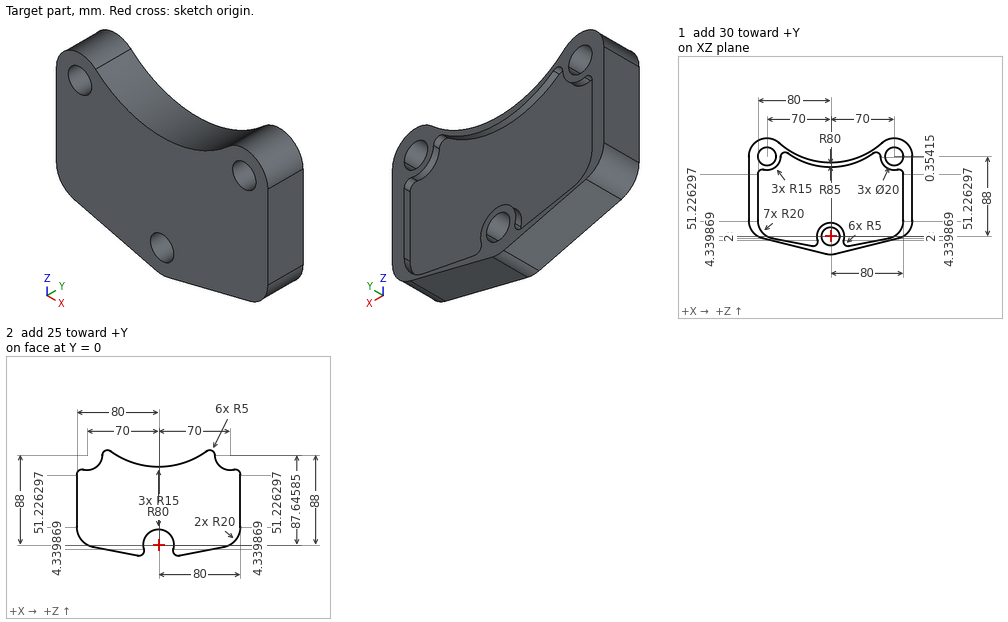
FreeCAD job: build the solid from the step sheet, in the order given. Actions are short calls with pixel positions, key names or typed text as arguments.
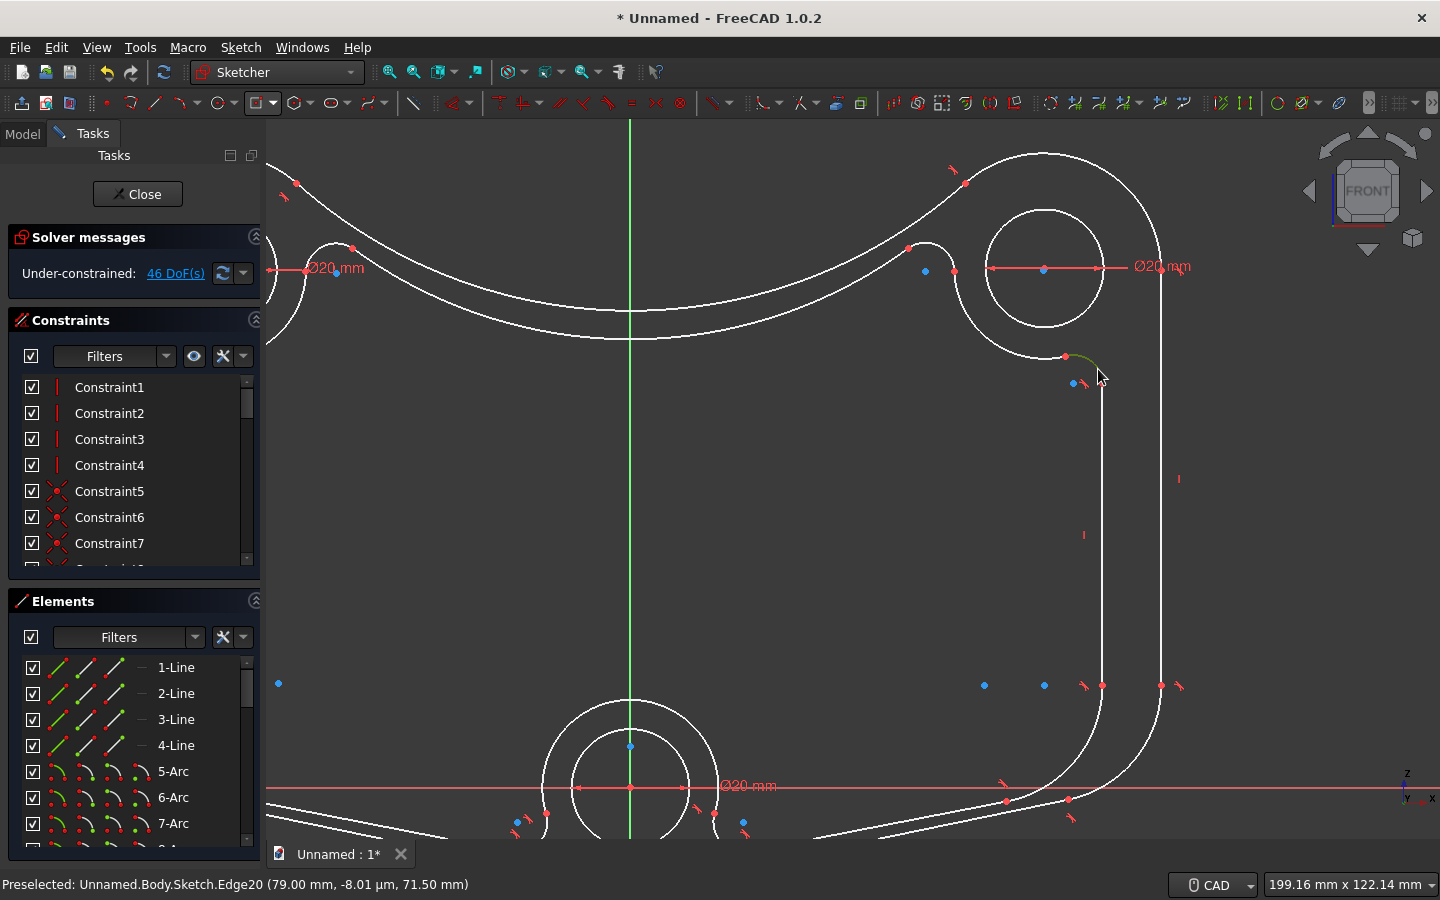
click(968, 317)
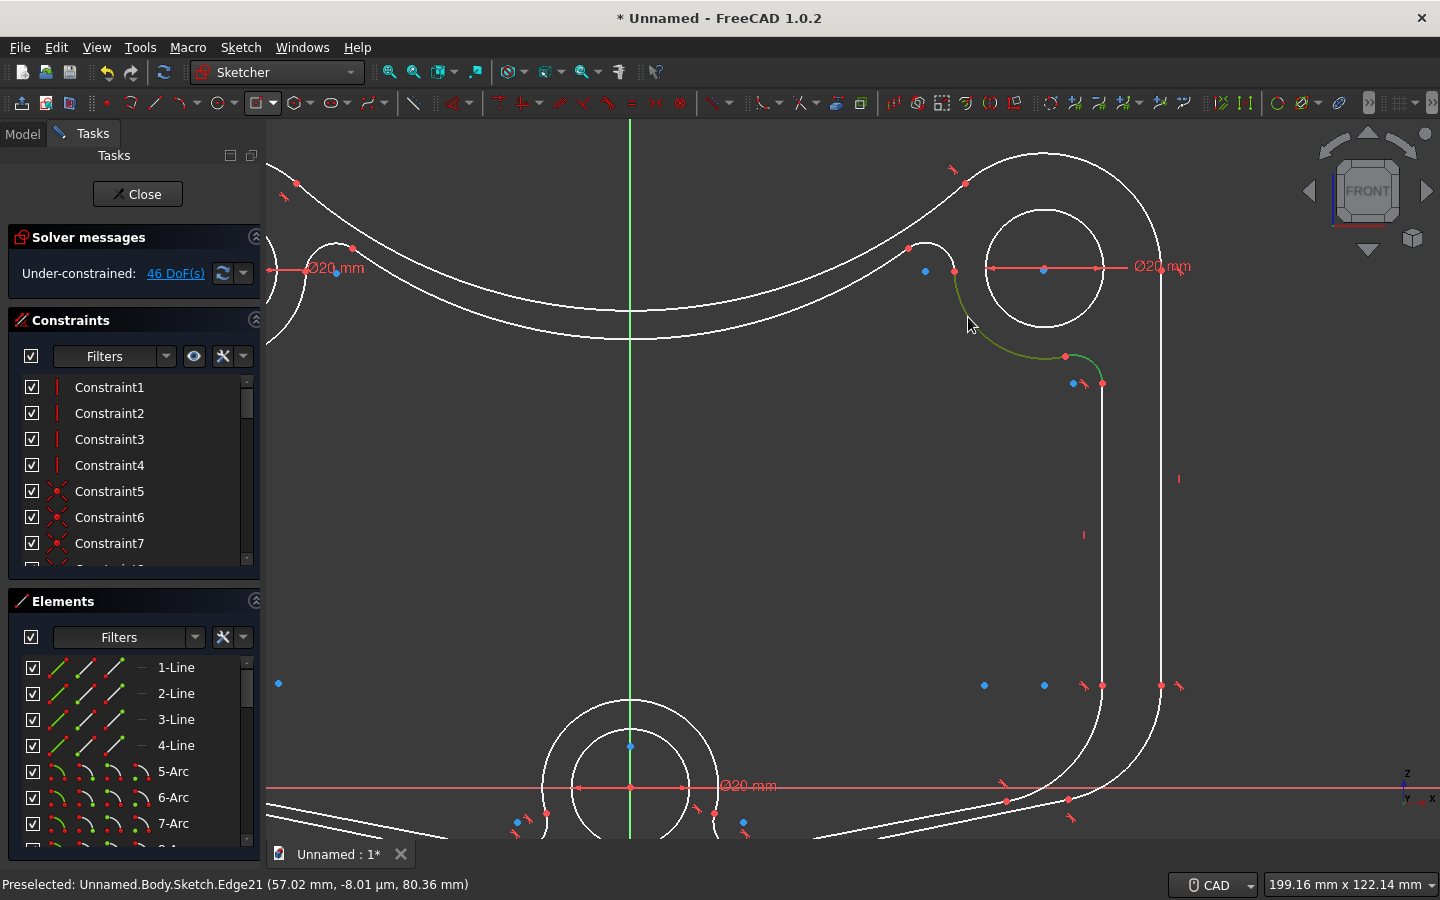
click(608, 104)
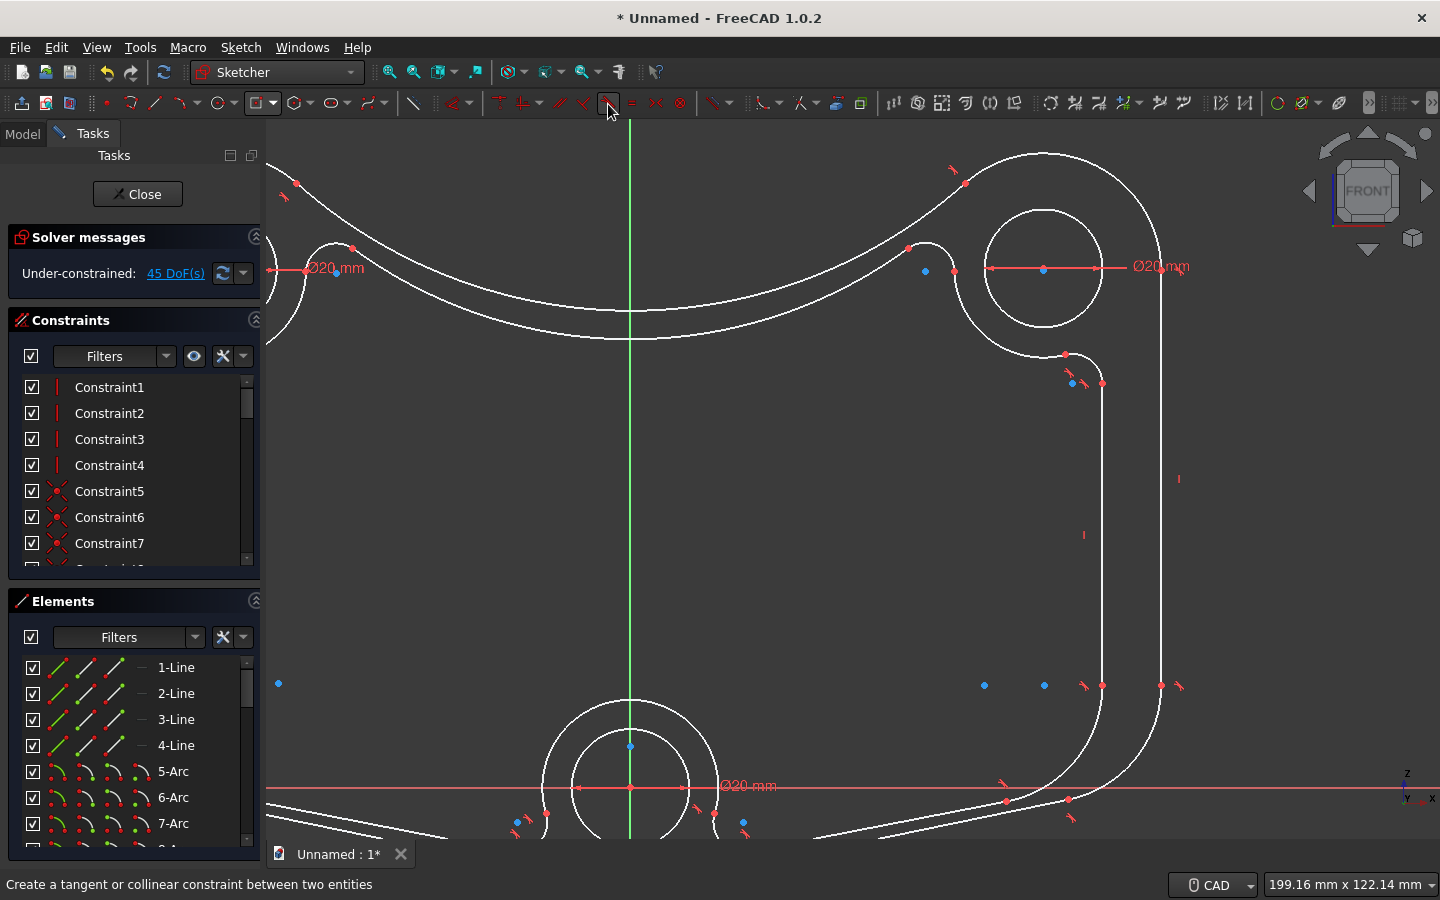
click(968, 316)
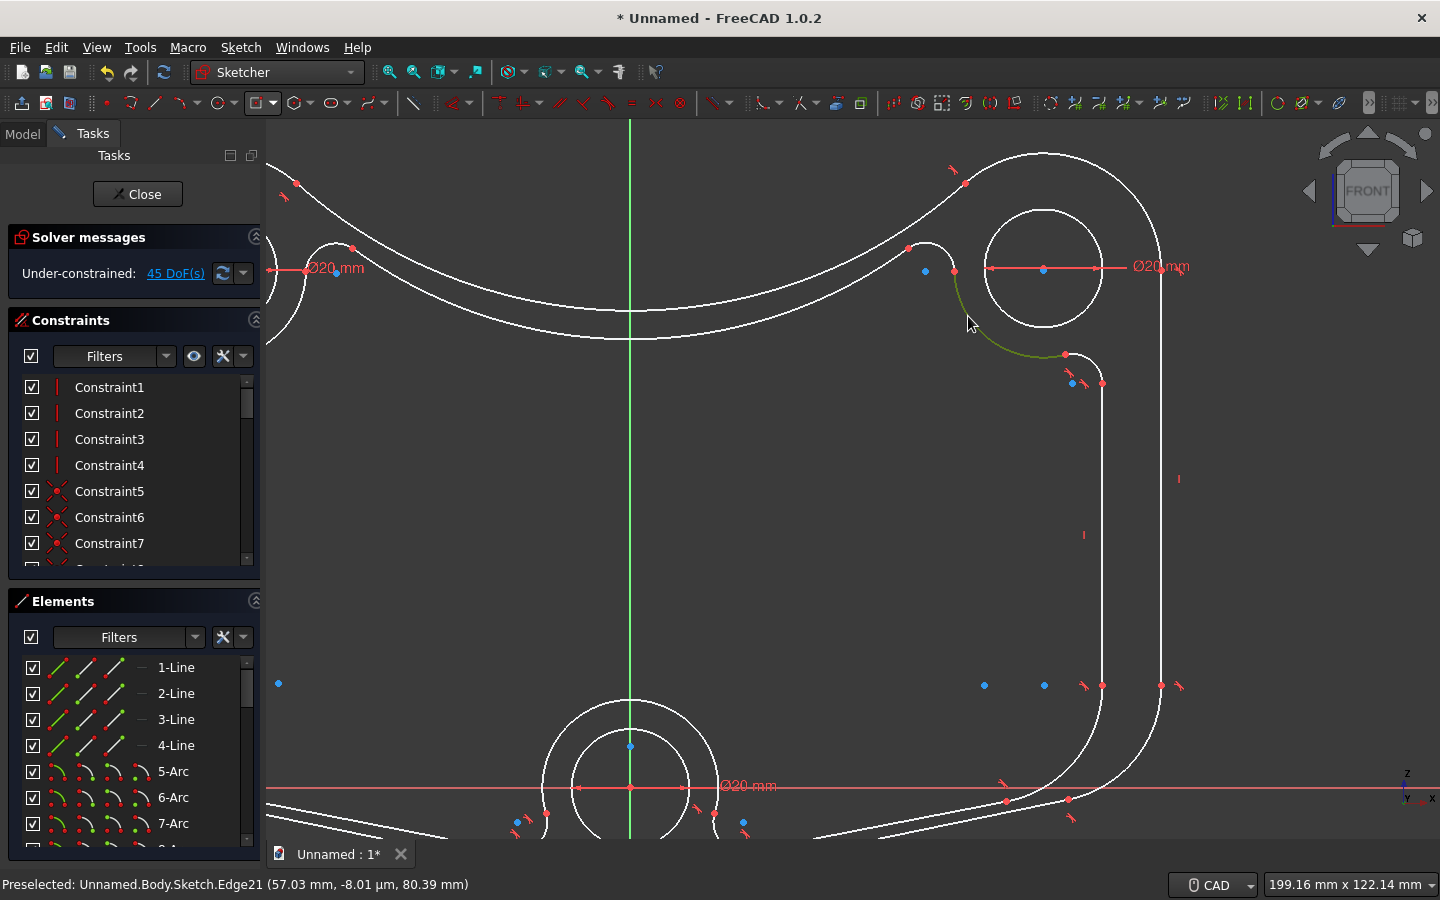
click(948, 254)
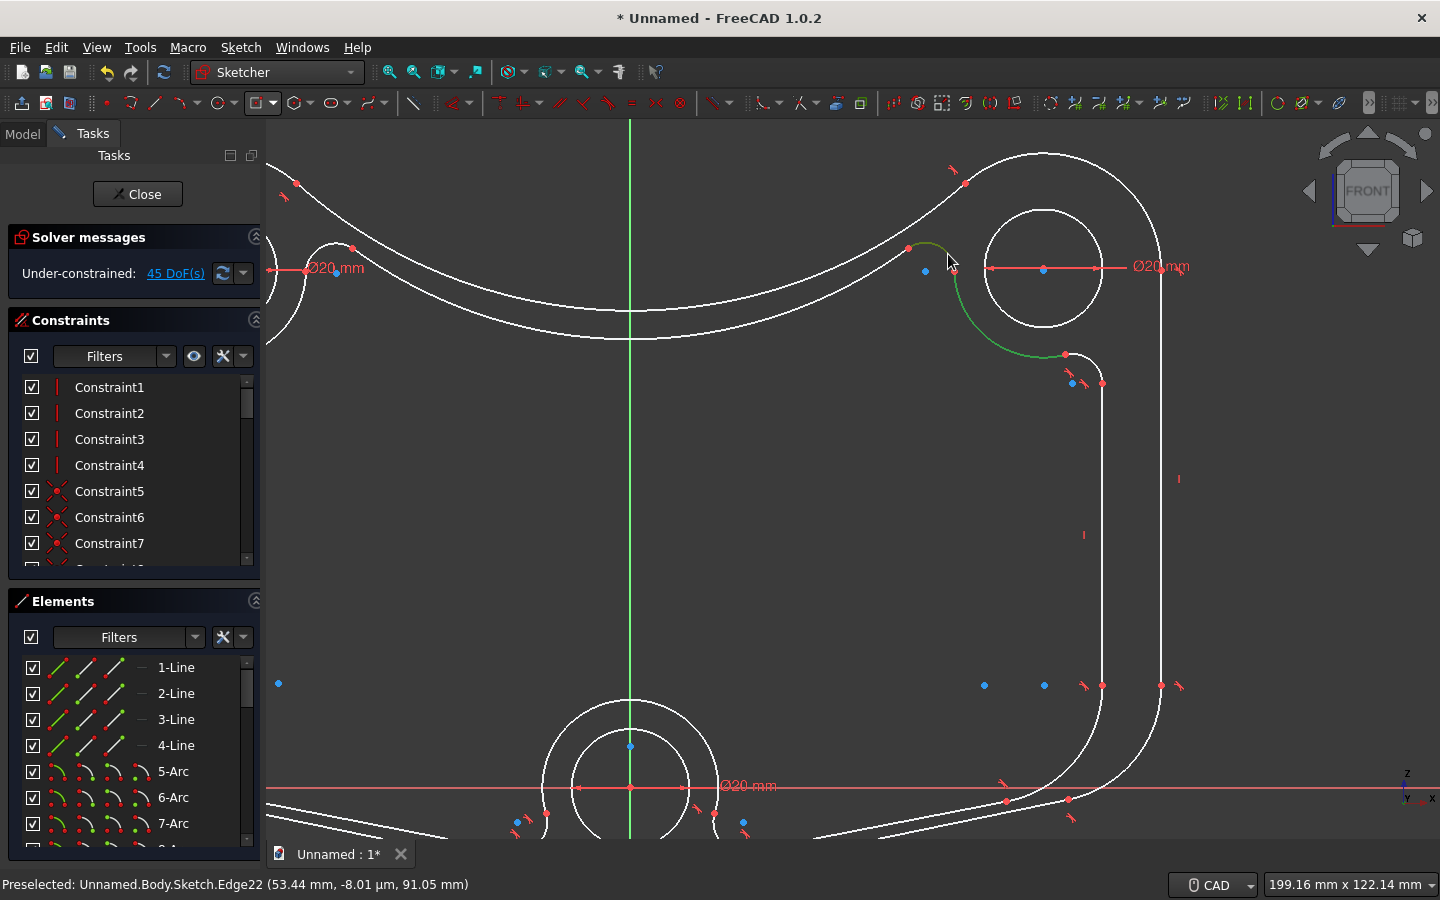
key(t)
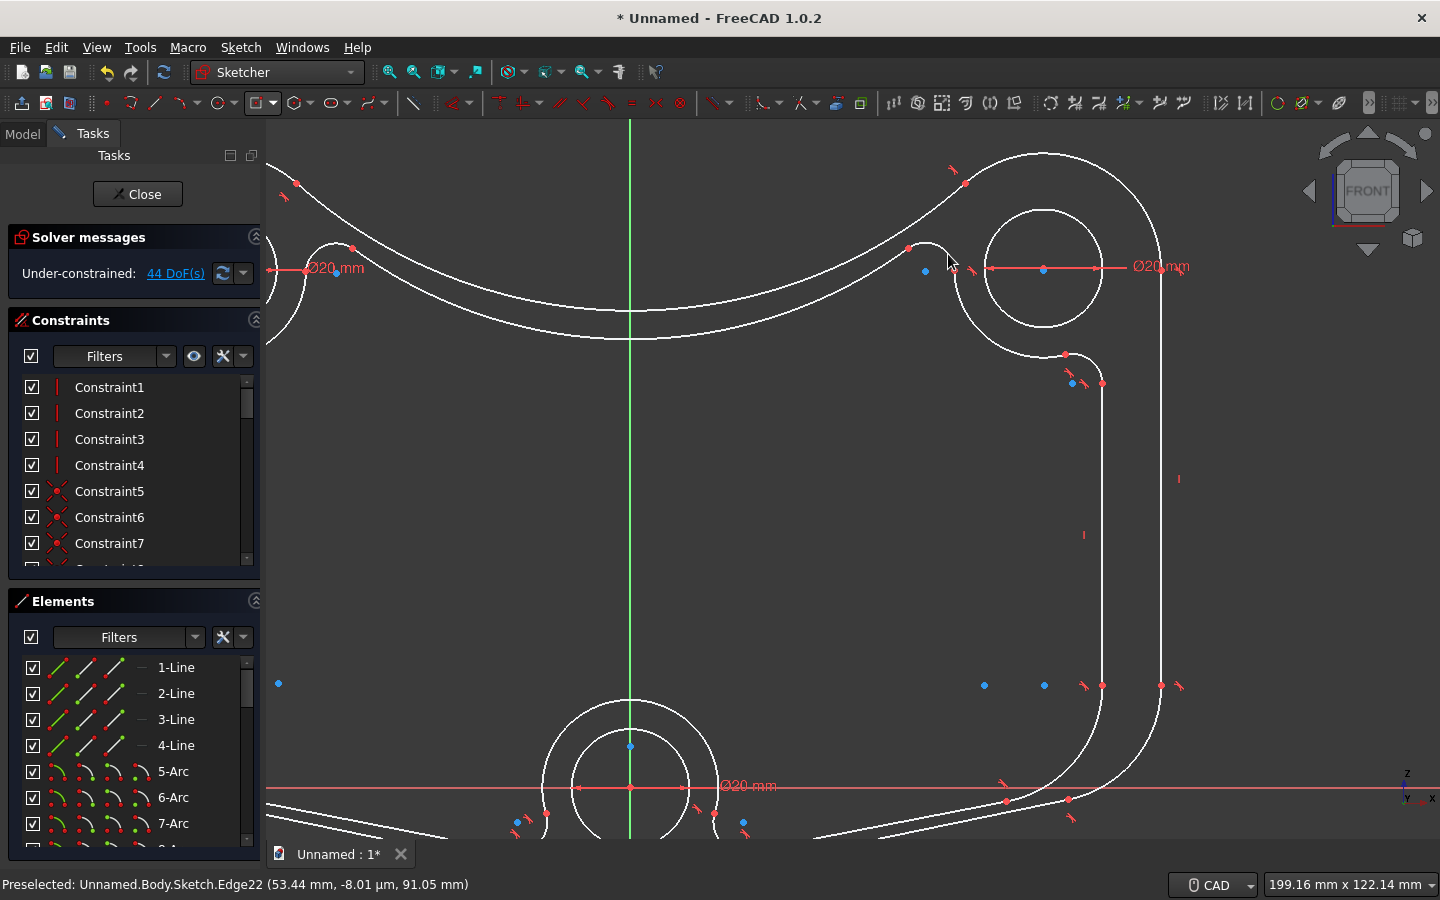
click(948, 253)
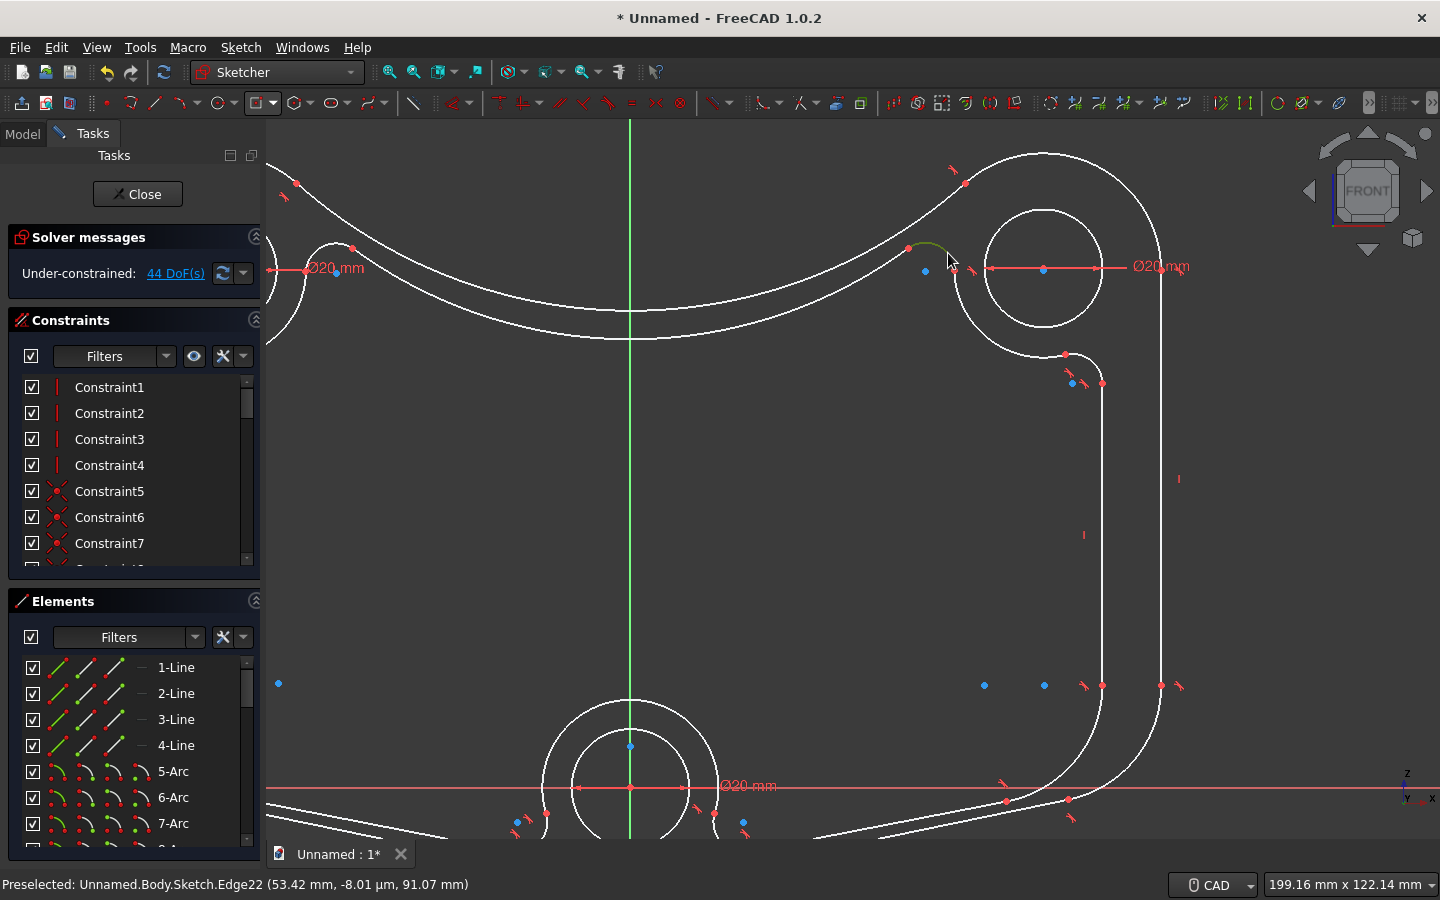
click(513, 324)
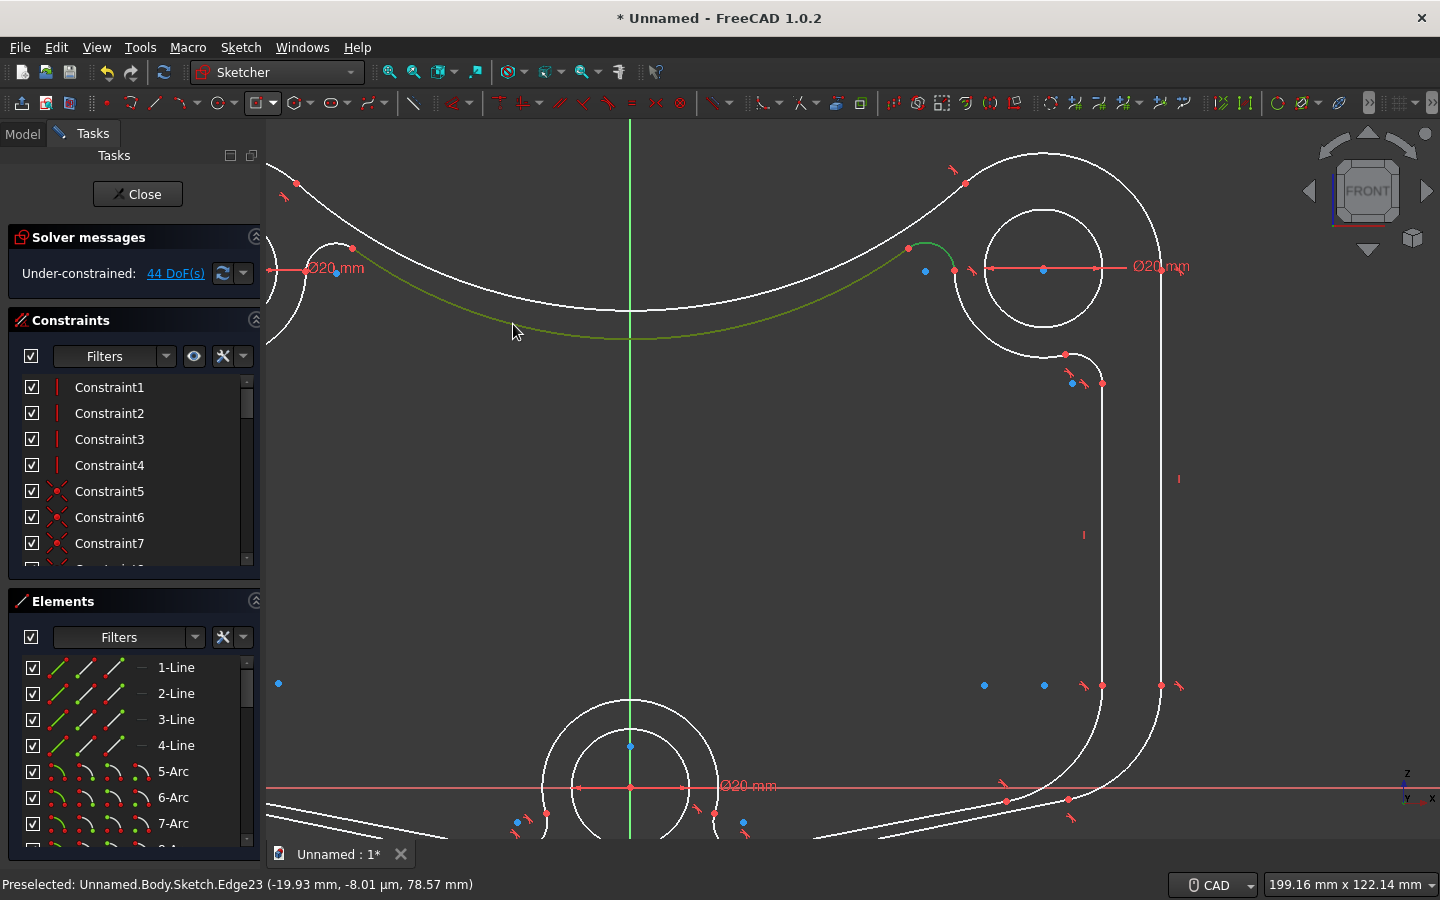
key(t)